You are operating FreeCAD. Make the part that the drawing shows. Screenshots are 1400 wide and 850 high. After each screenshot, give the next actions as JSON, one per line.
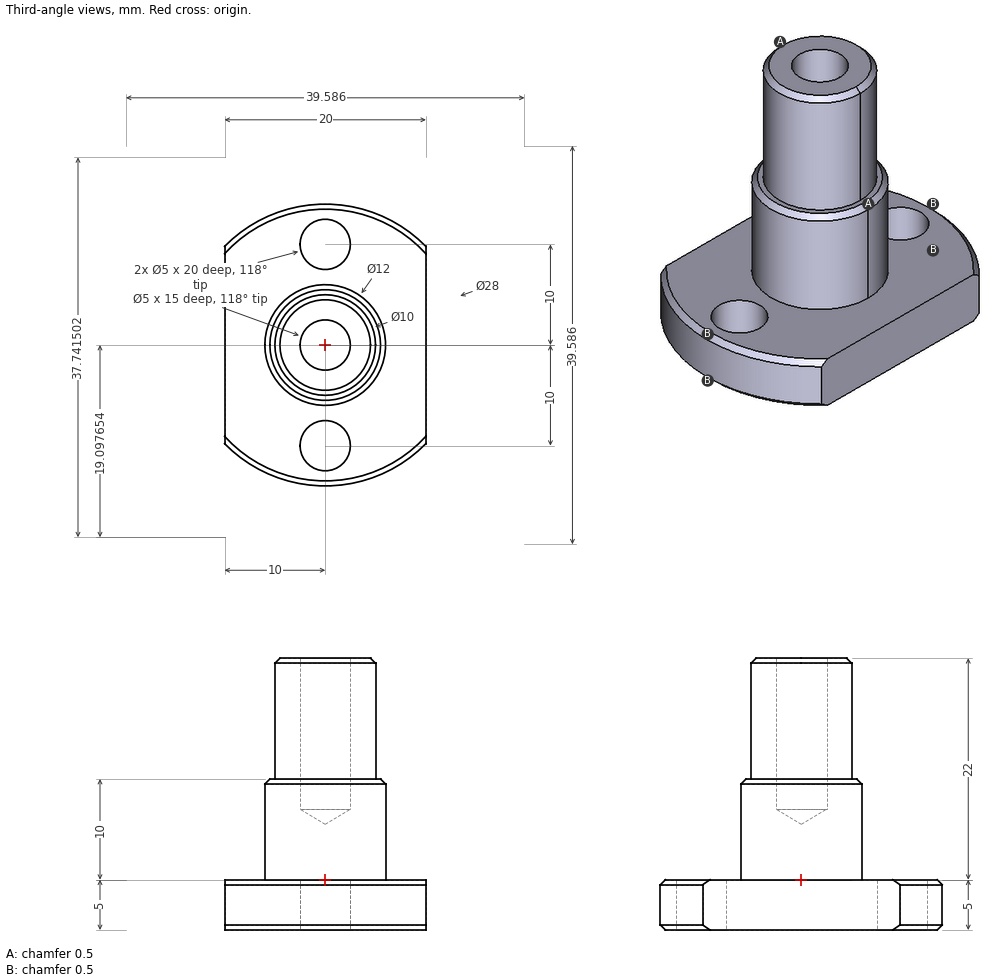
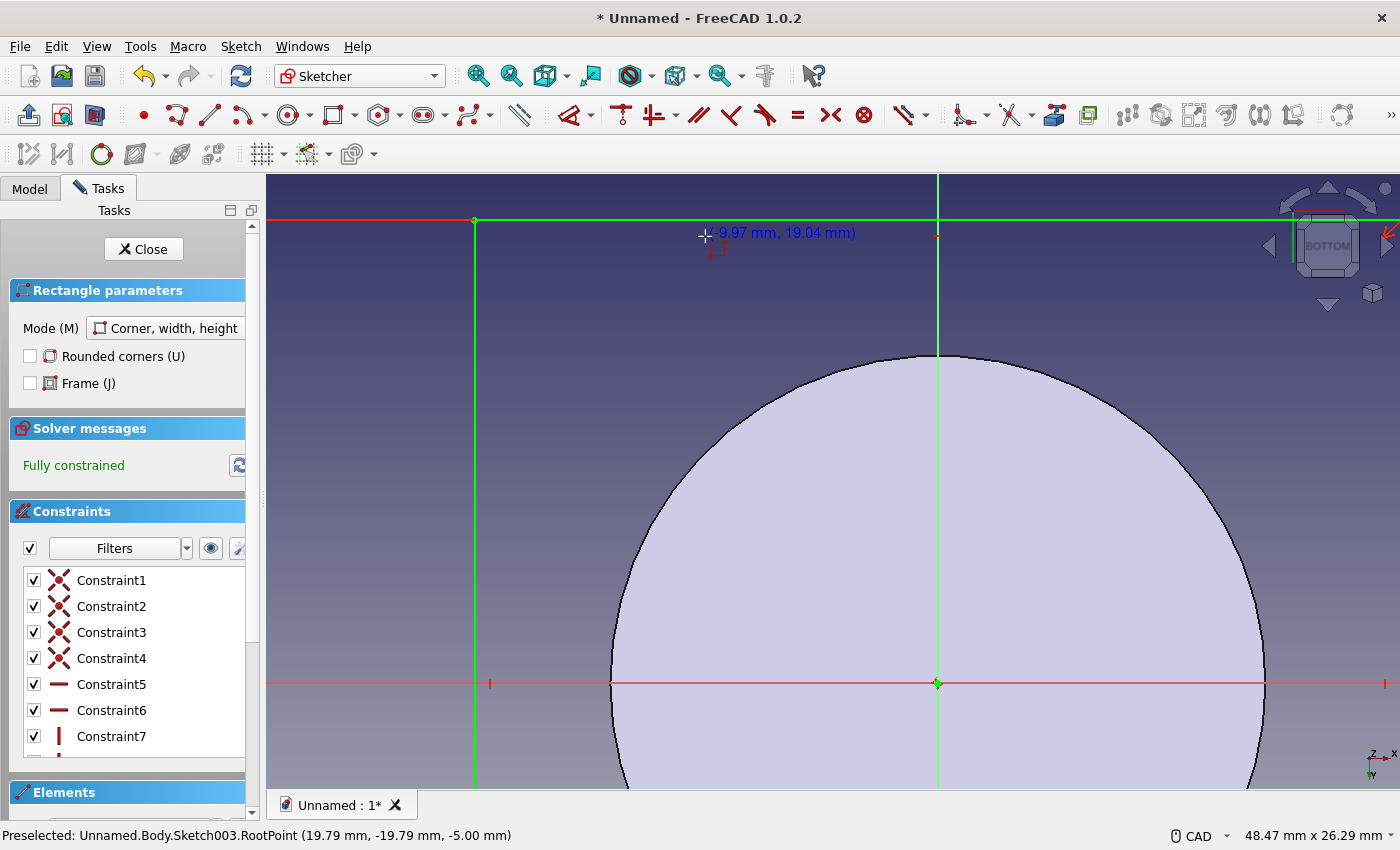
{"action": "left_click", "coordinate": [704, 236]}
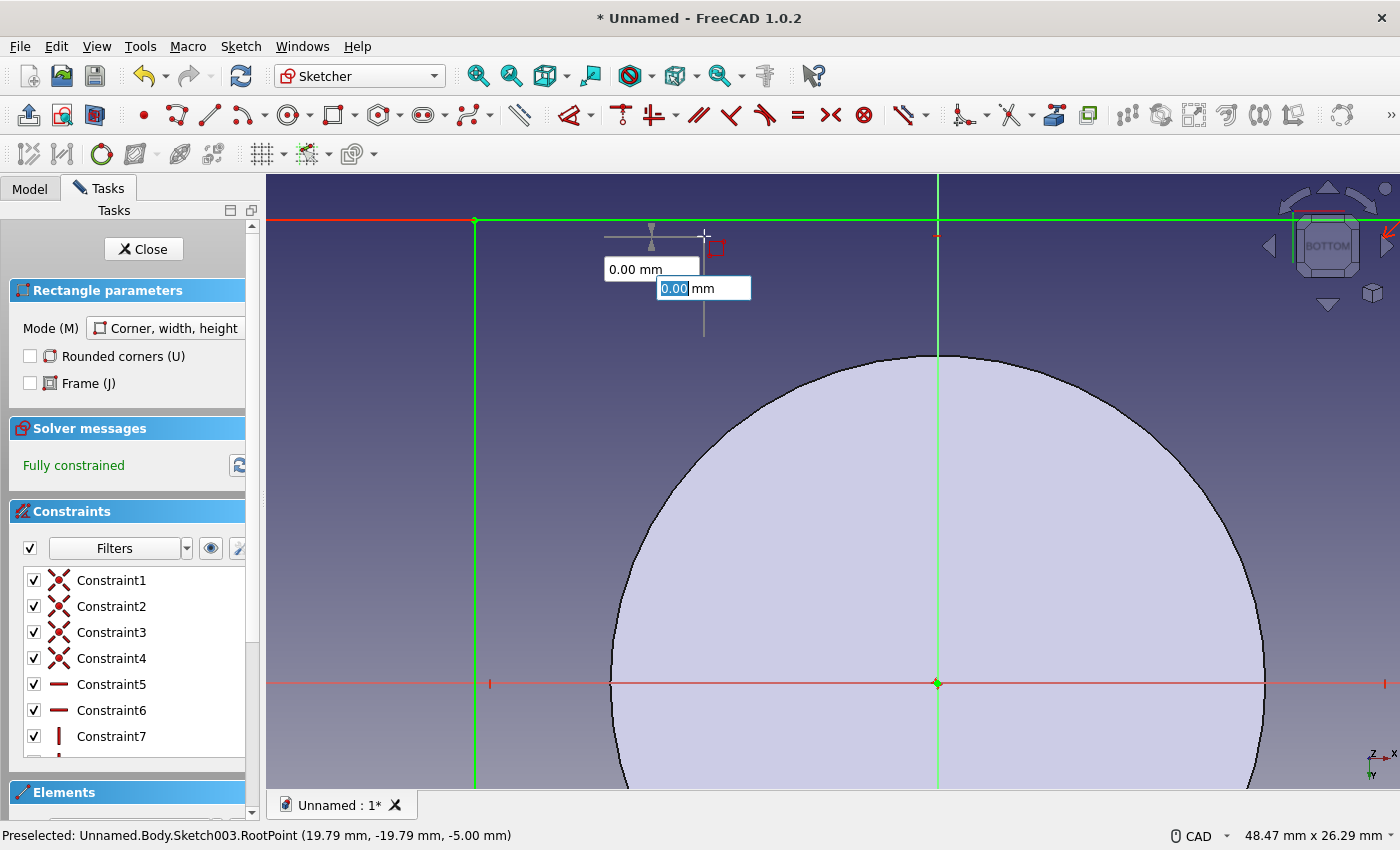
{"action": "scroll", "coordinate": [623, 317], "scroll_direction": "down", "scroll_amount": 4}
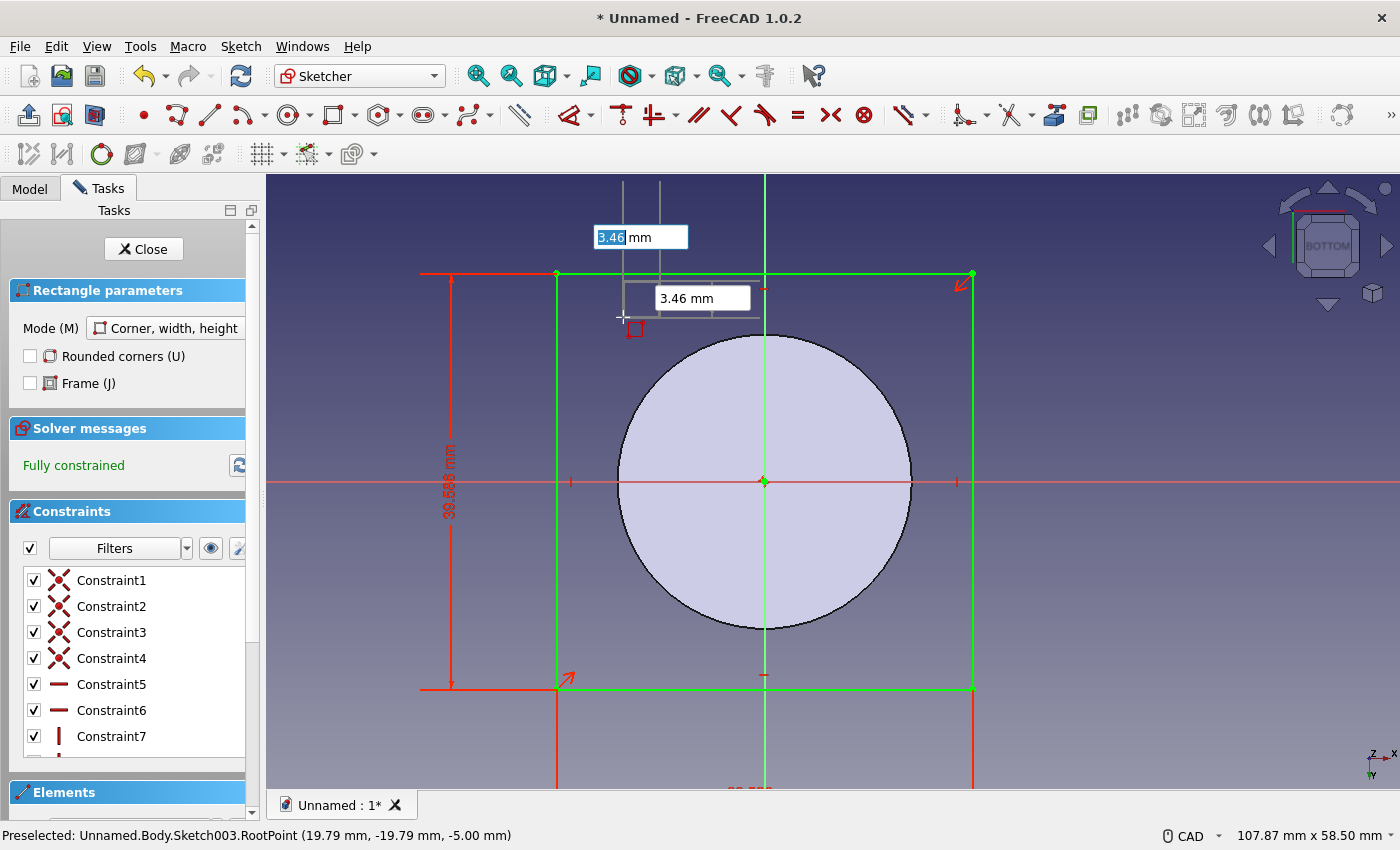
{"action": "scroll", "coordinate": [870, 678], "scroll_direction": "up", "scroll_amount": 2}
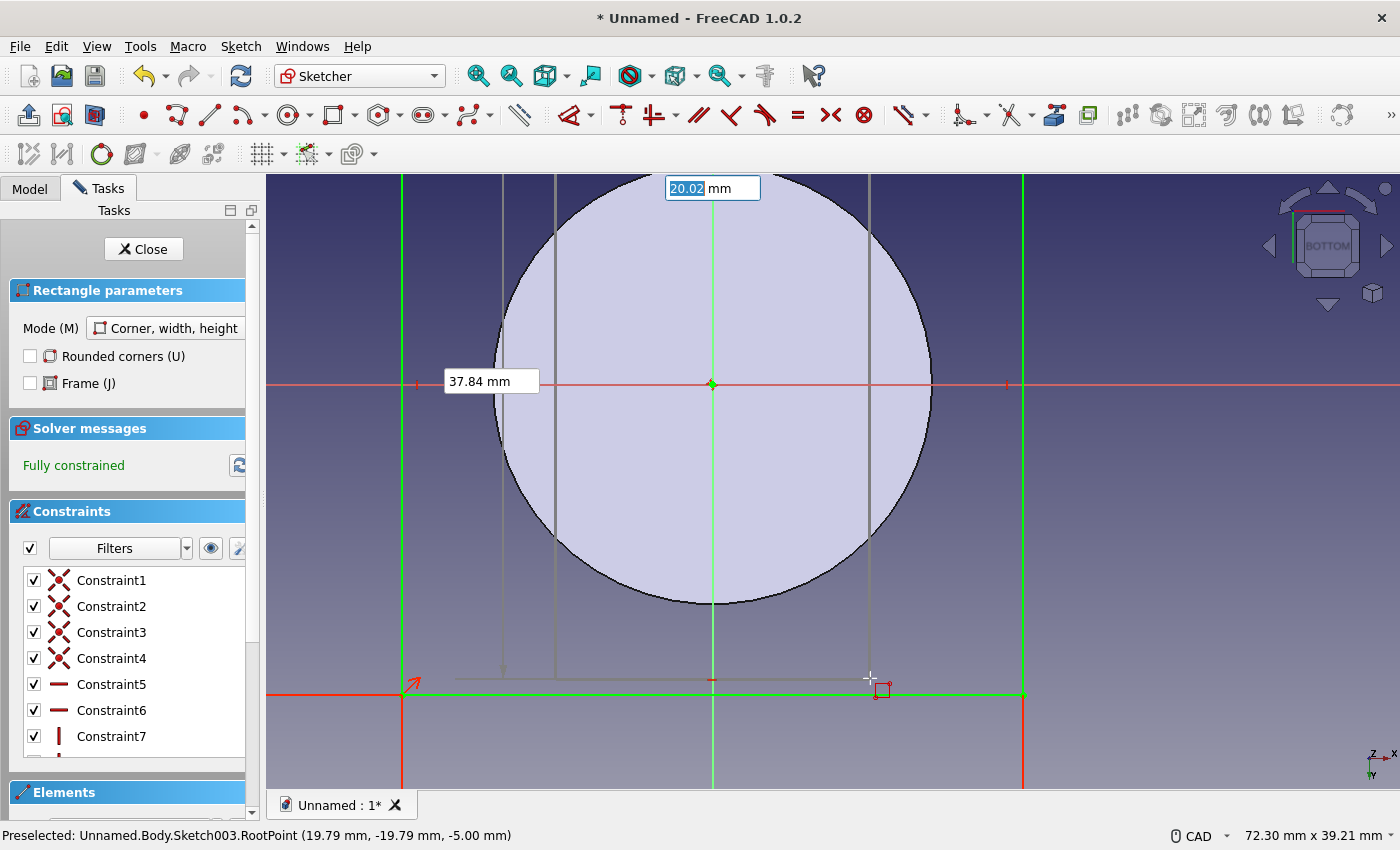
{"action": "left_click", "coordinate": [869, 677]}
{"action": "key", "text": "Escape"}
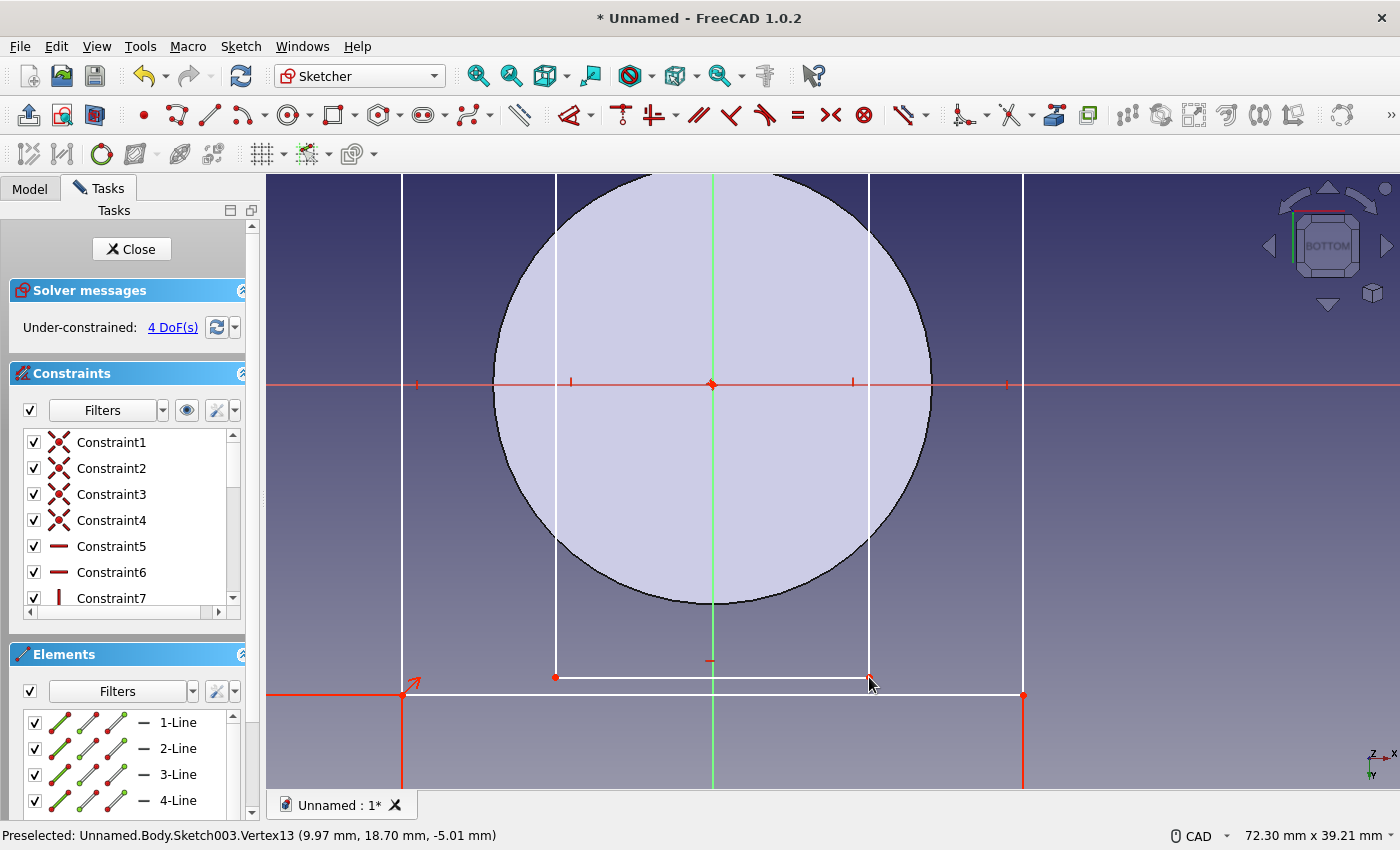
{"action": "left_click", "coordinate": [650, 678]}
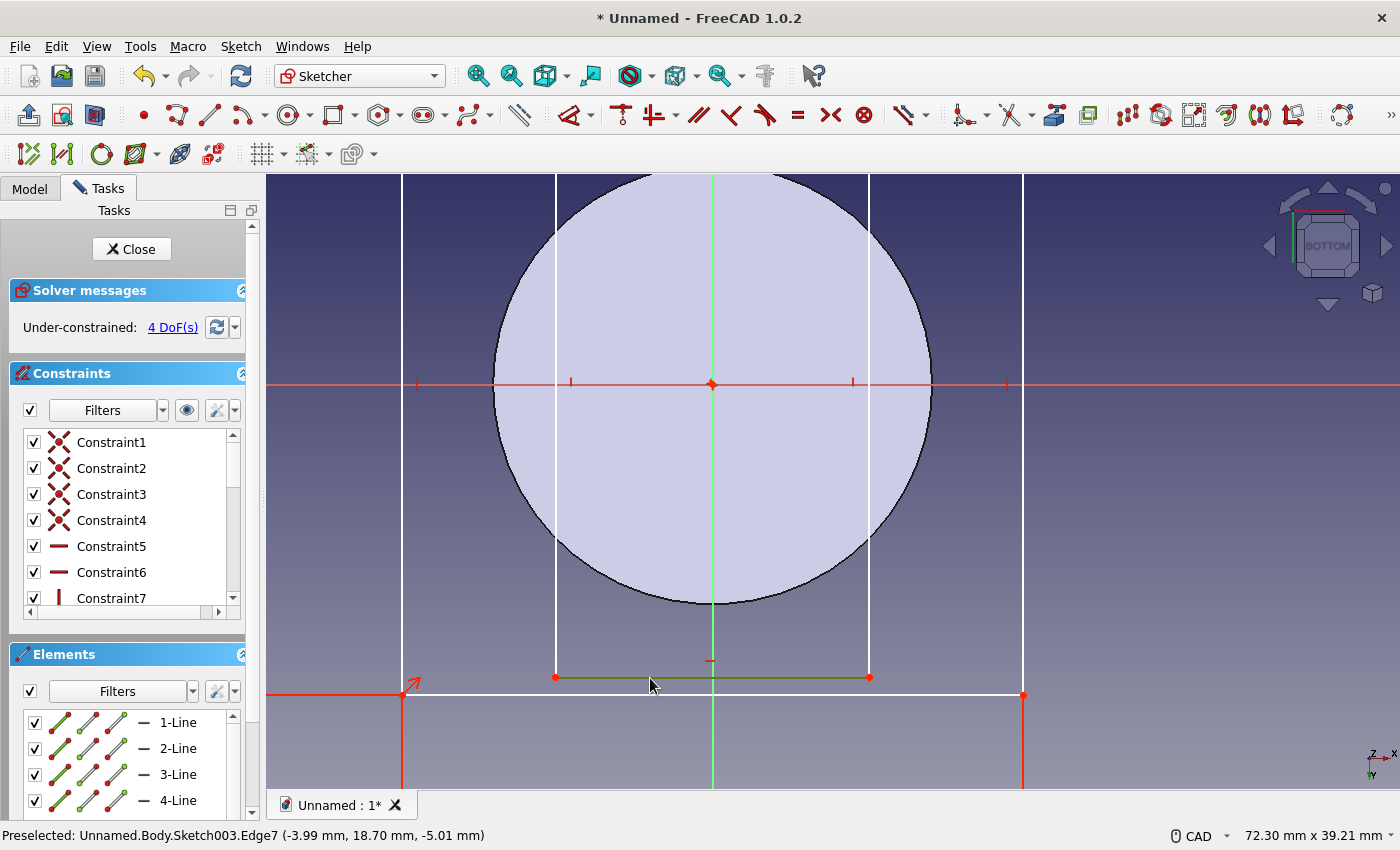
{"action": "key", "text": "l"}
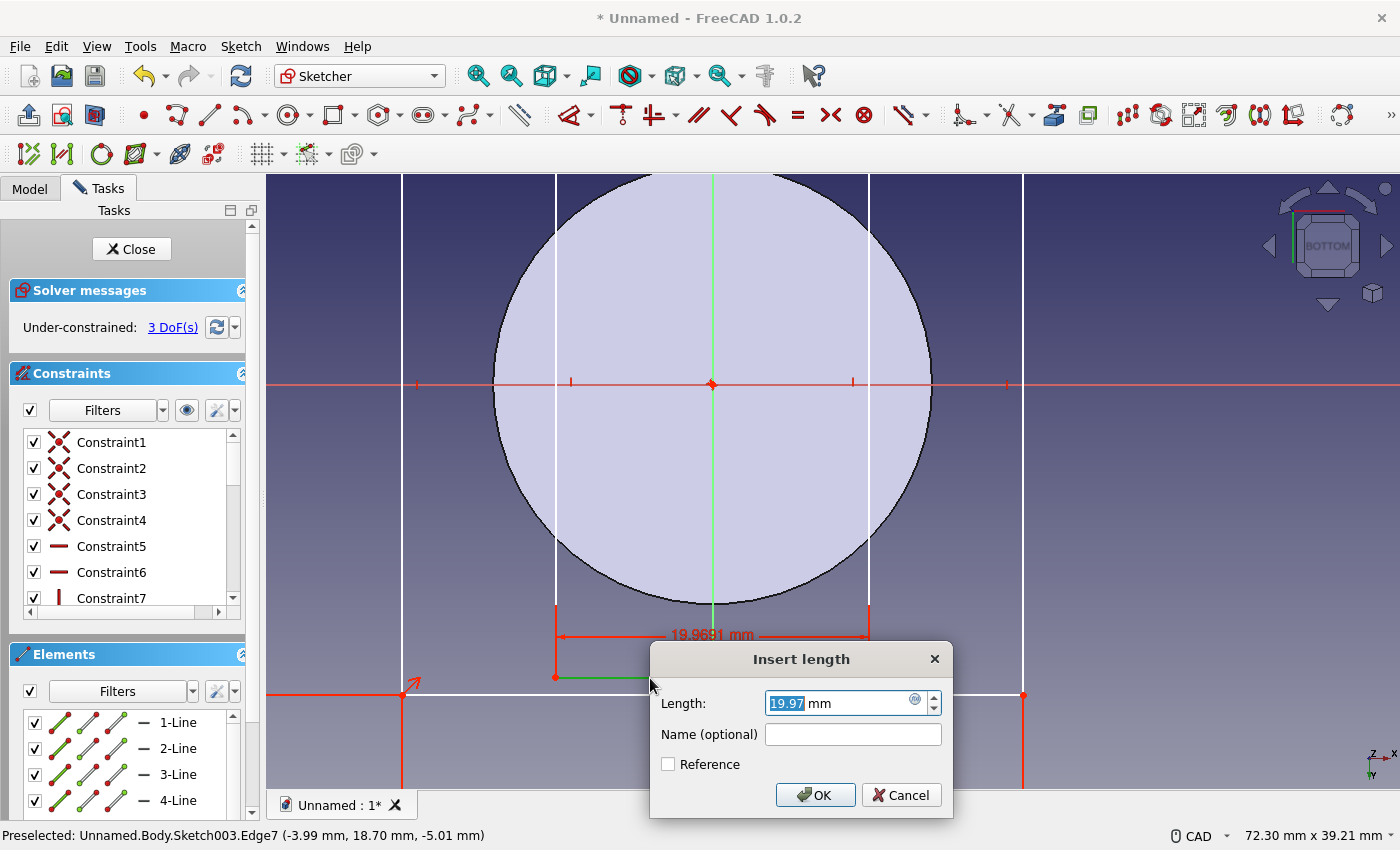
{"action": "type", "text": "20"}
{"action": "key", "text": "Return"}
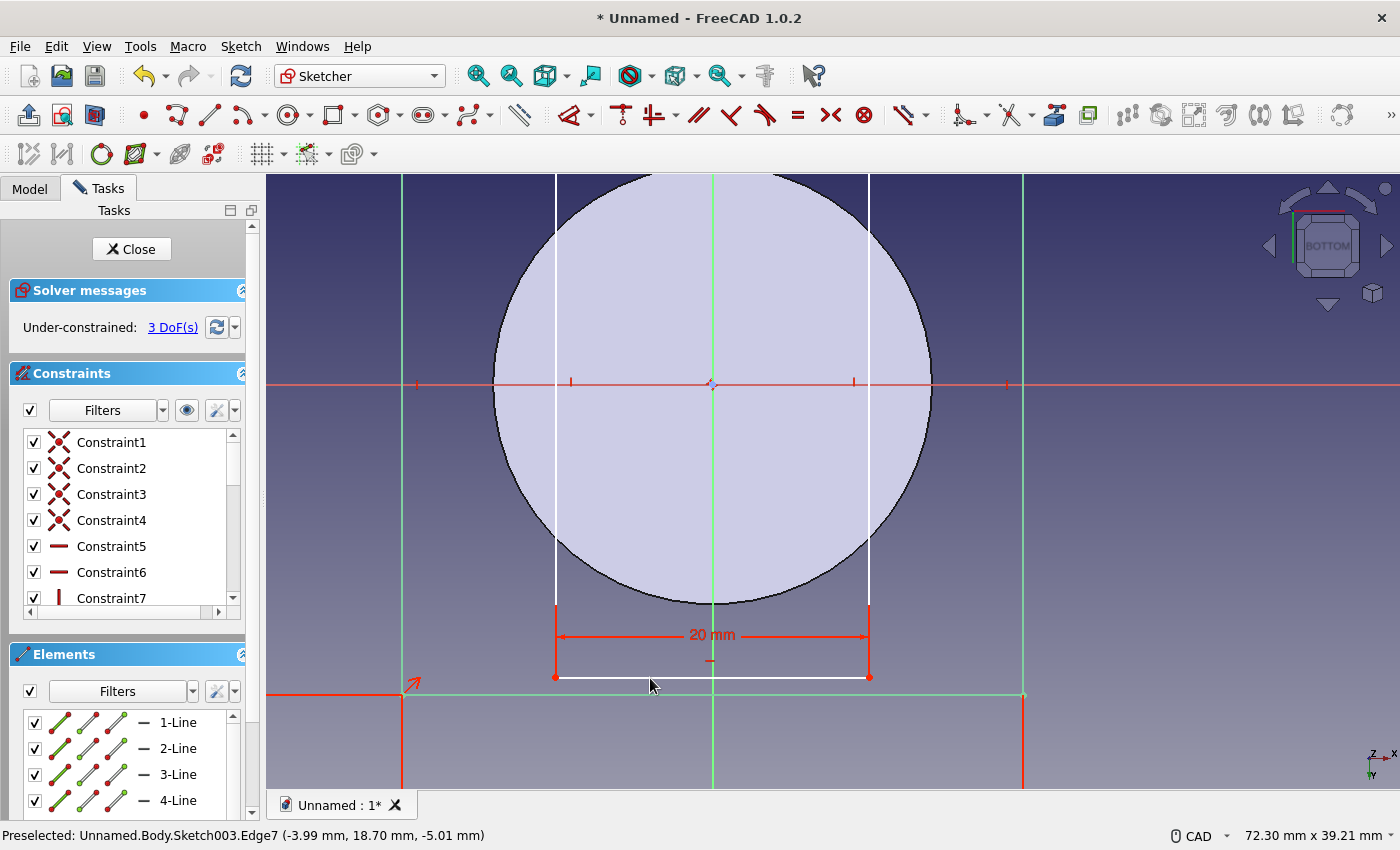
{"action": "scroll", "coordinate": [870, 678], "scroll_direction": "down", "scroll_amount": 2}